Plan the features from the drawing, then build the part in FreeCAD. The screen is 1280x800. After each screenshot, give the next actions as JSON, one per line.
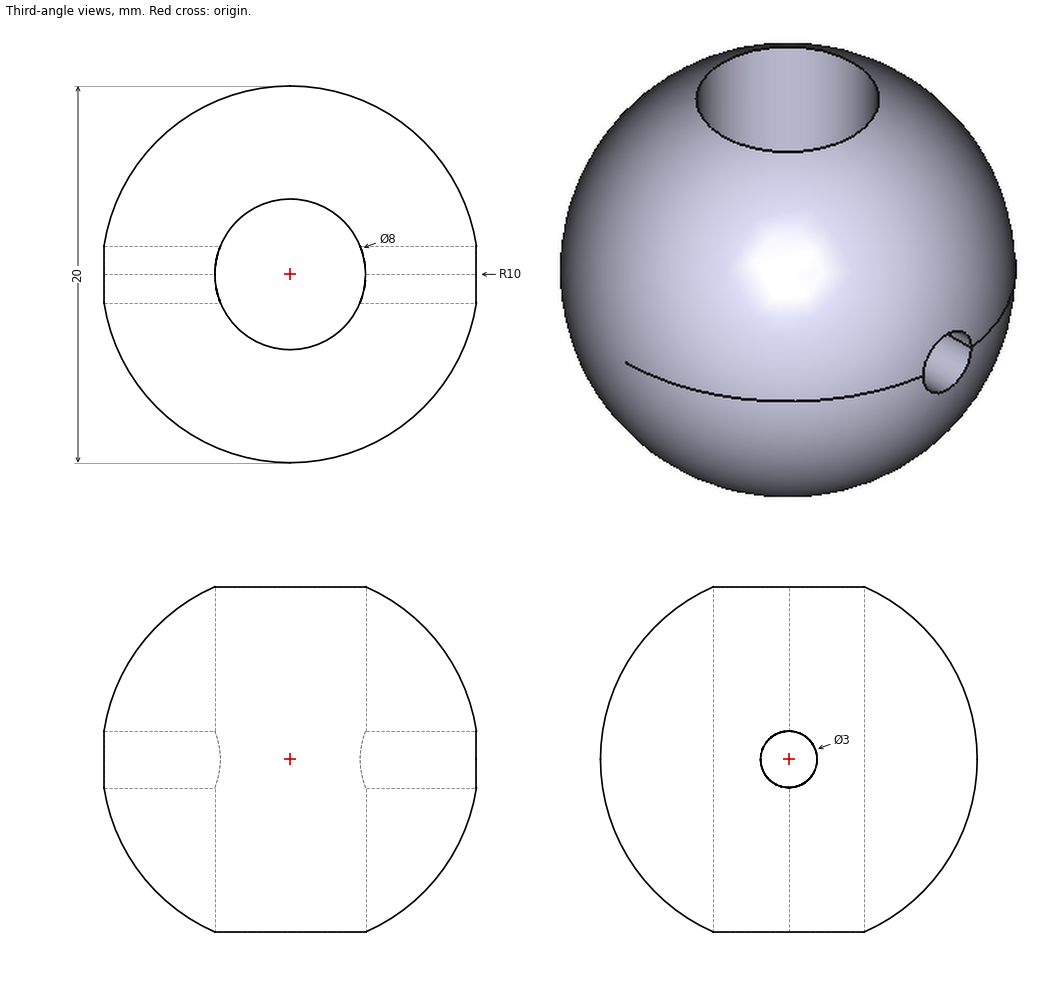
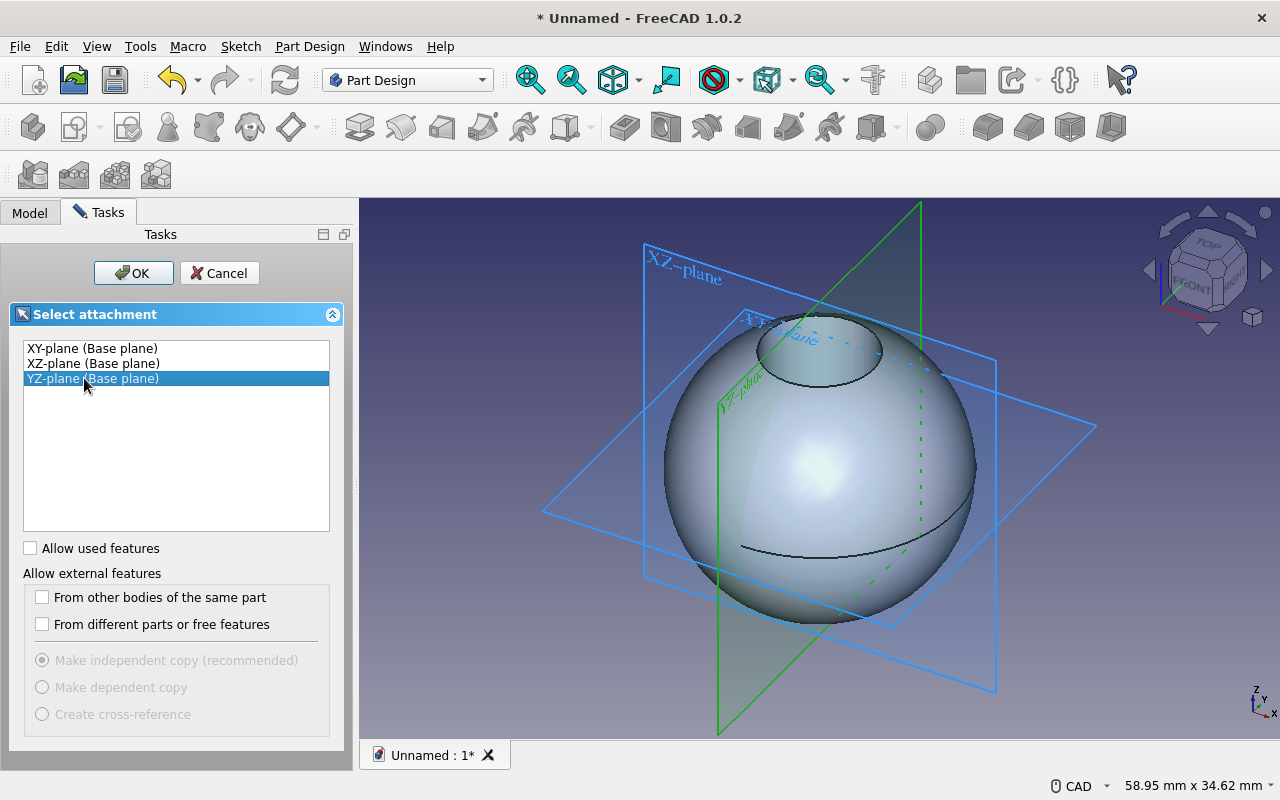
{"action": "left_click", "coordinate": [134, 273]}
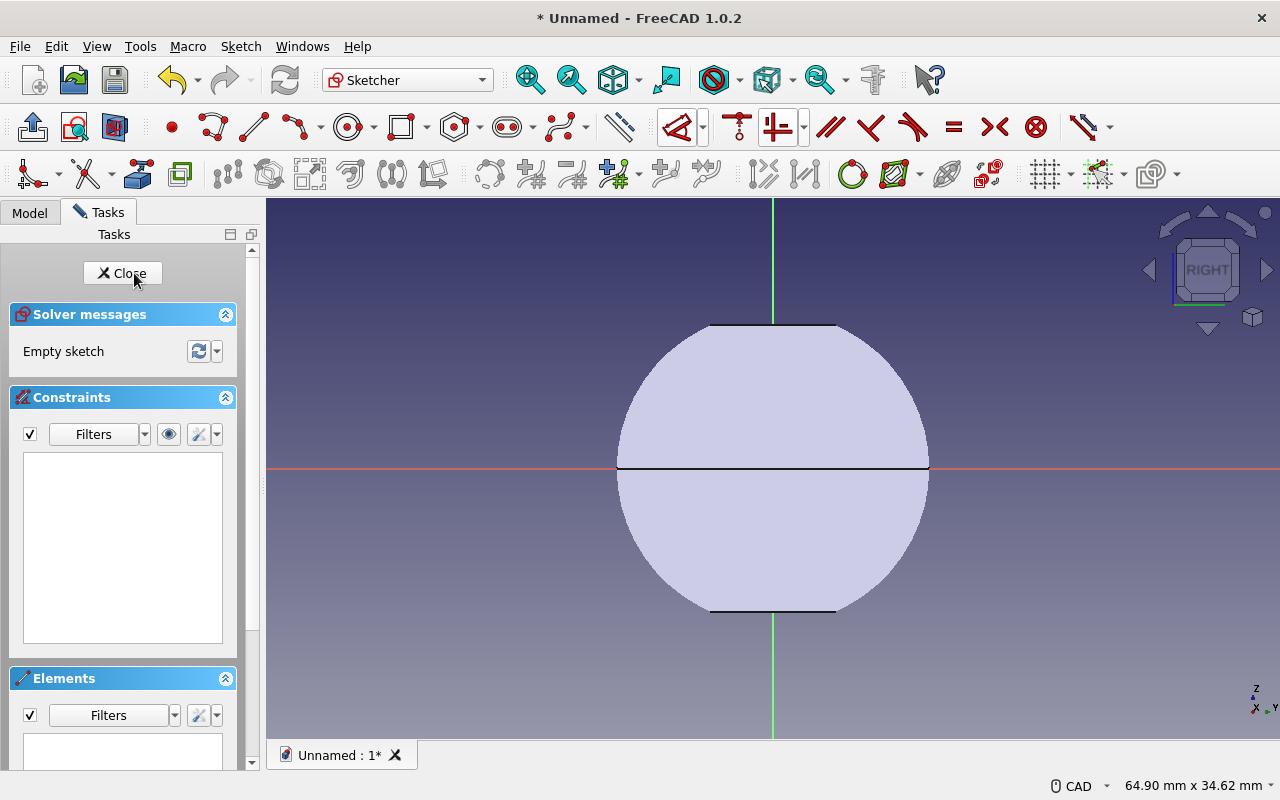
{"action": "left_click", "coordinate": [115, 128]}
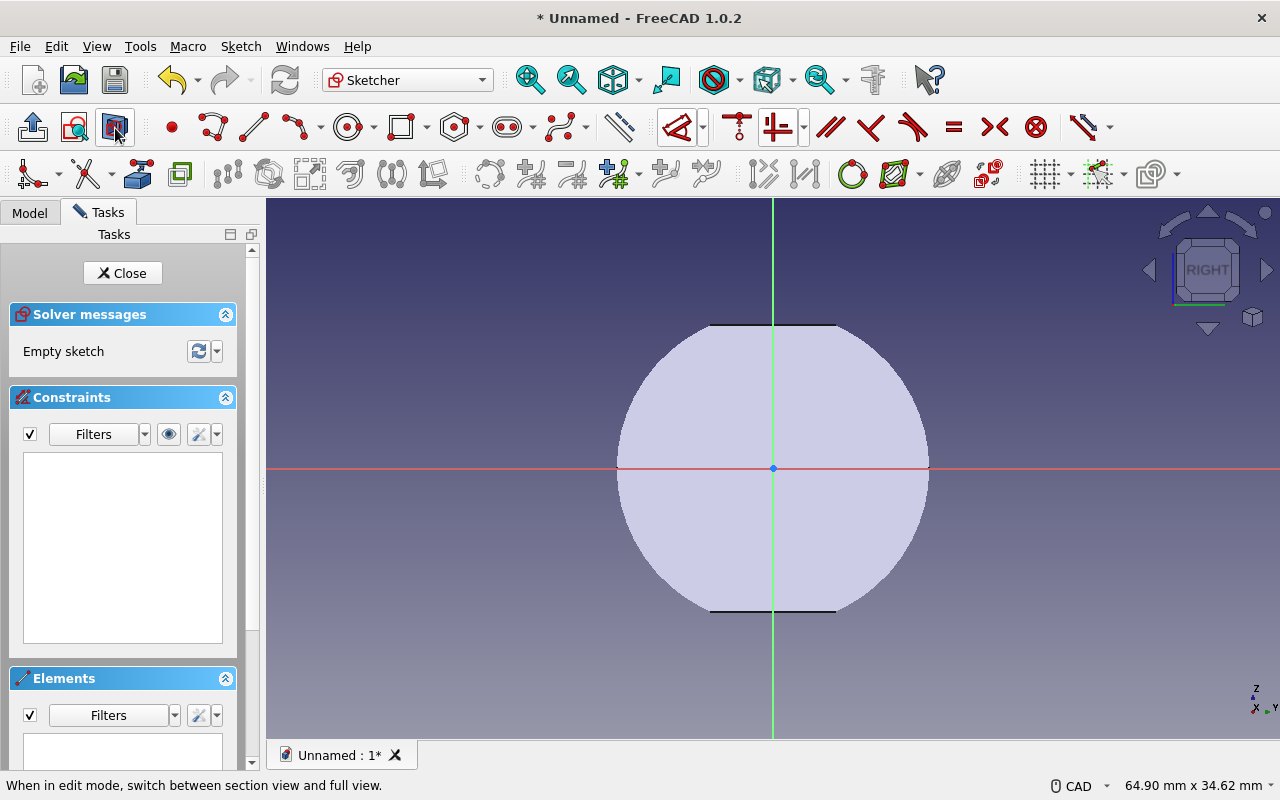
{"action": "scroll", "coordinate": [784, 468], "scroll_direction": "up", "scroll_amount": 10}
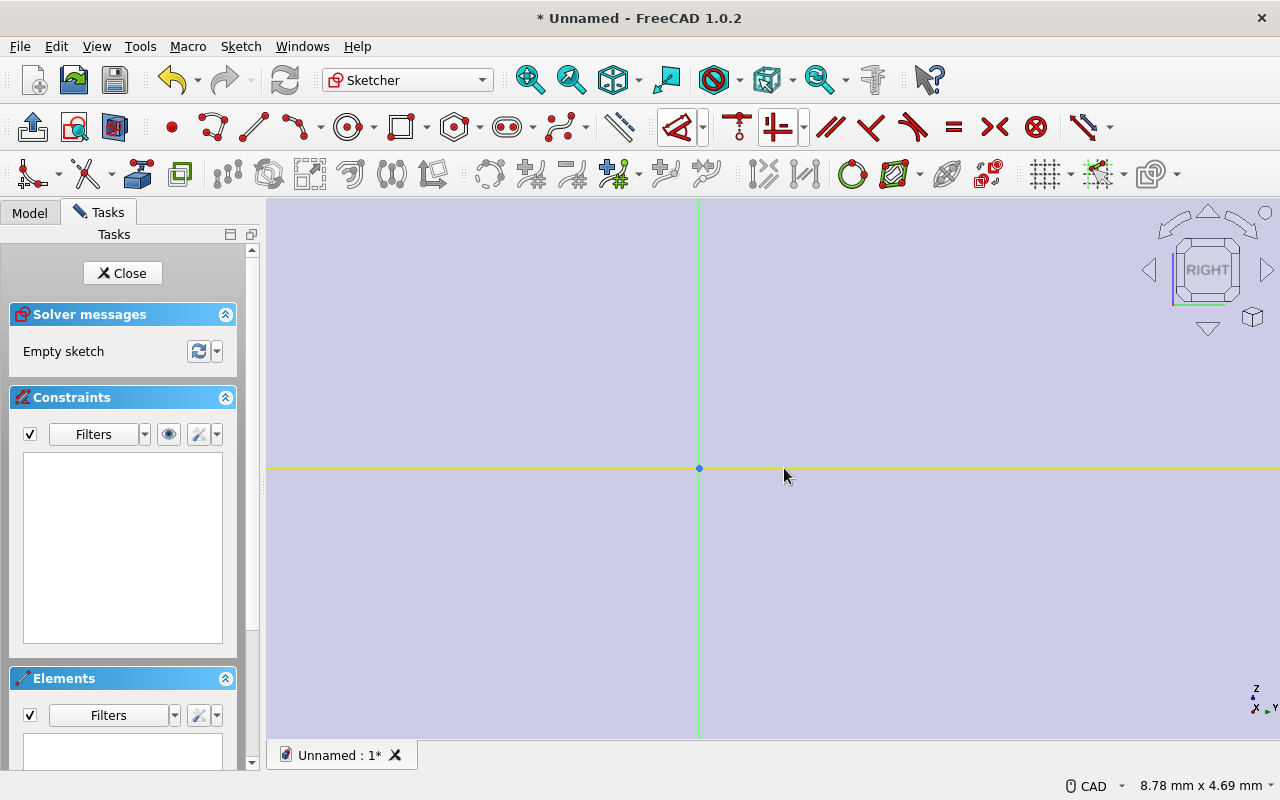
{"action": "left_click", "coordinate": [348, 128]}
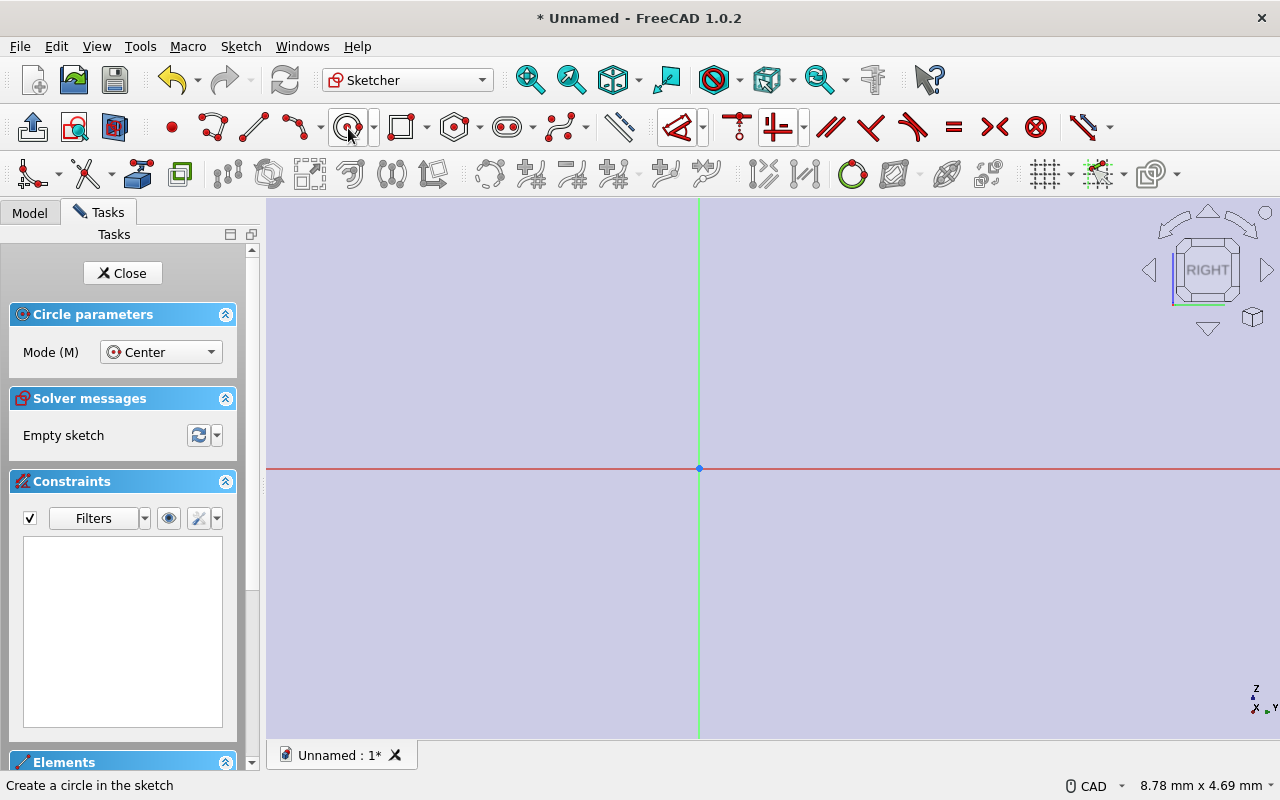
{"action": "left_click", "coordinate": [699, 468]}
{"action": "mouse_move", "coordinate": [822, 346]}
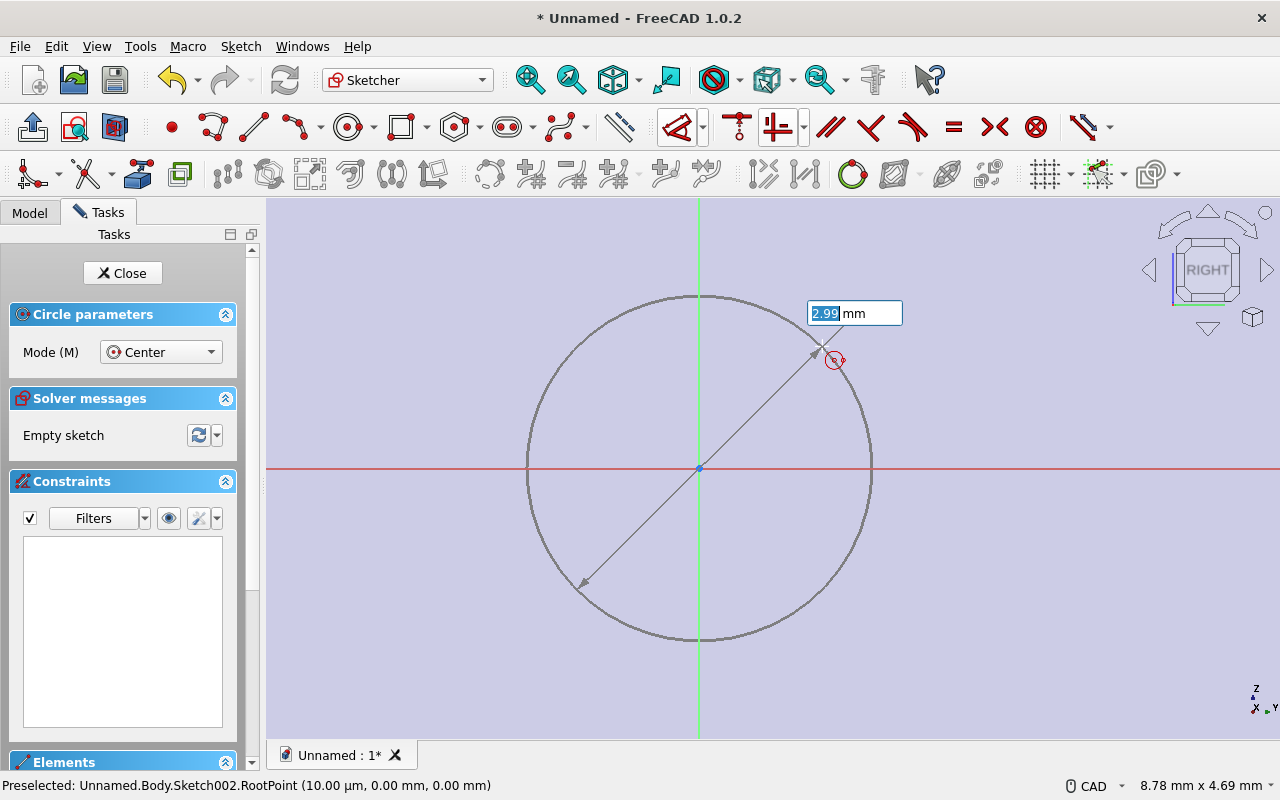
{"action": "type", "text": "3"}
{"action": "key", "text": "Return"}
{"action": "key", "text": "Escape"}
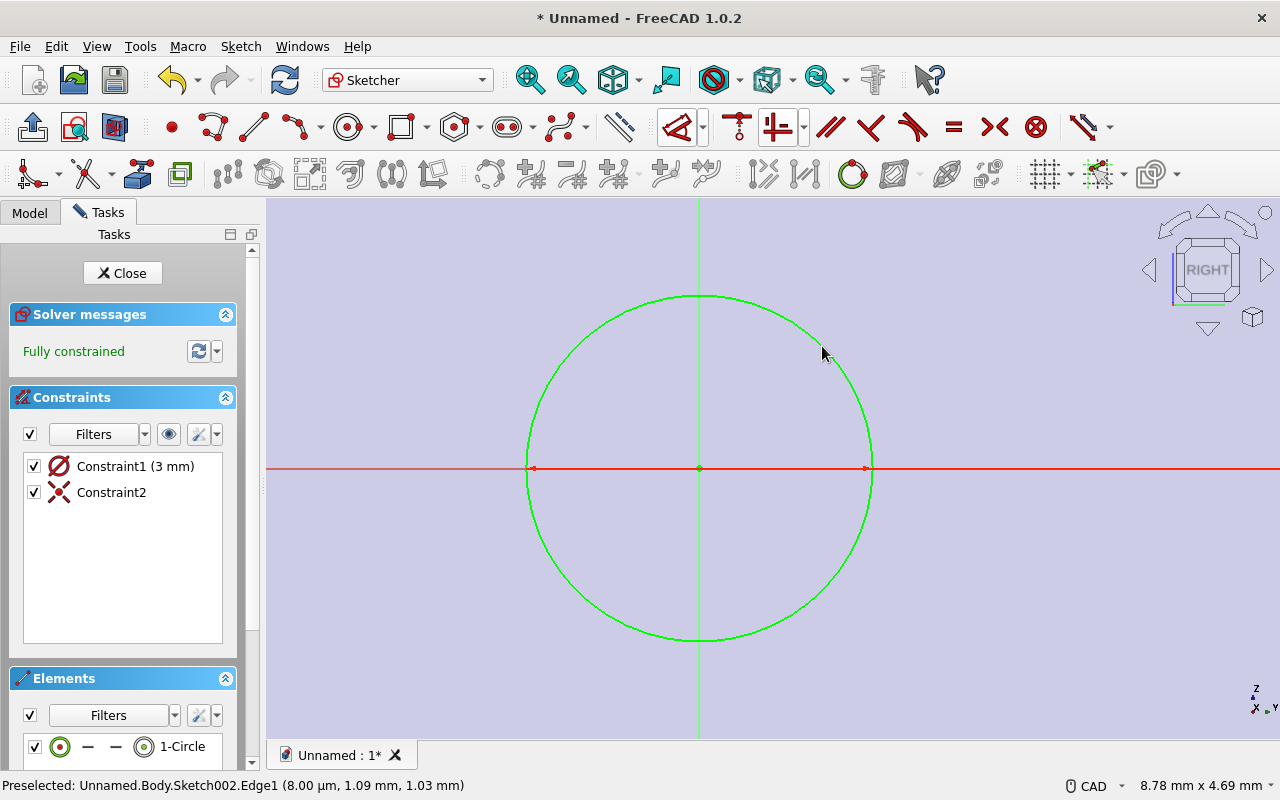
{"action": "left_click", "coordinate": [123, 273]}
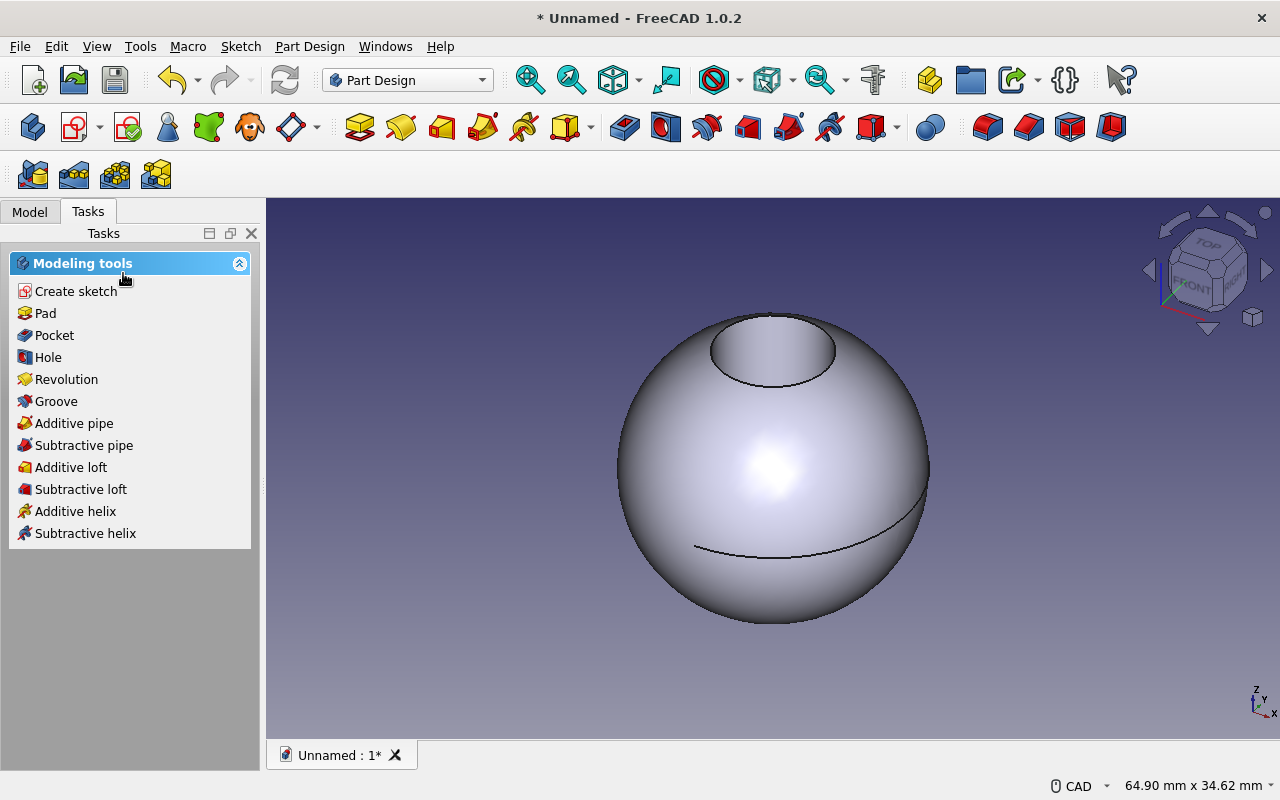
{"action": "left_click", "coordinate": [625, 128]}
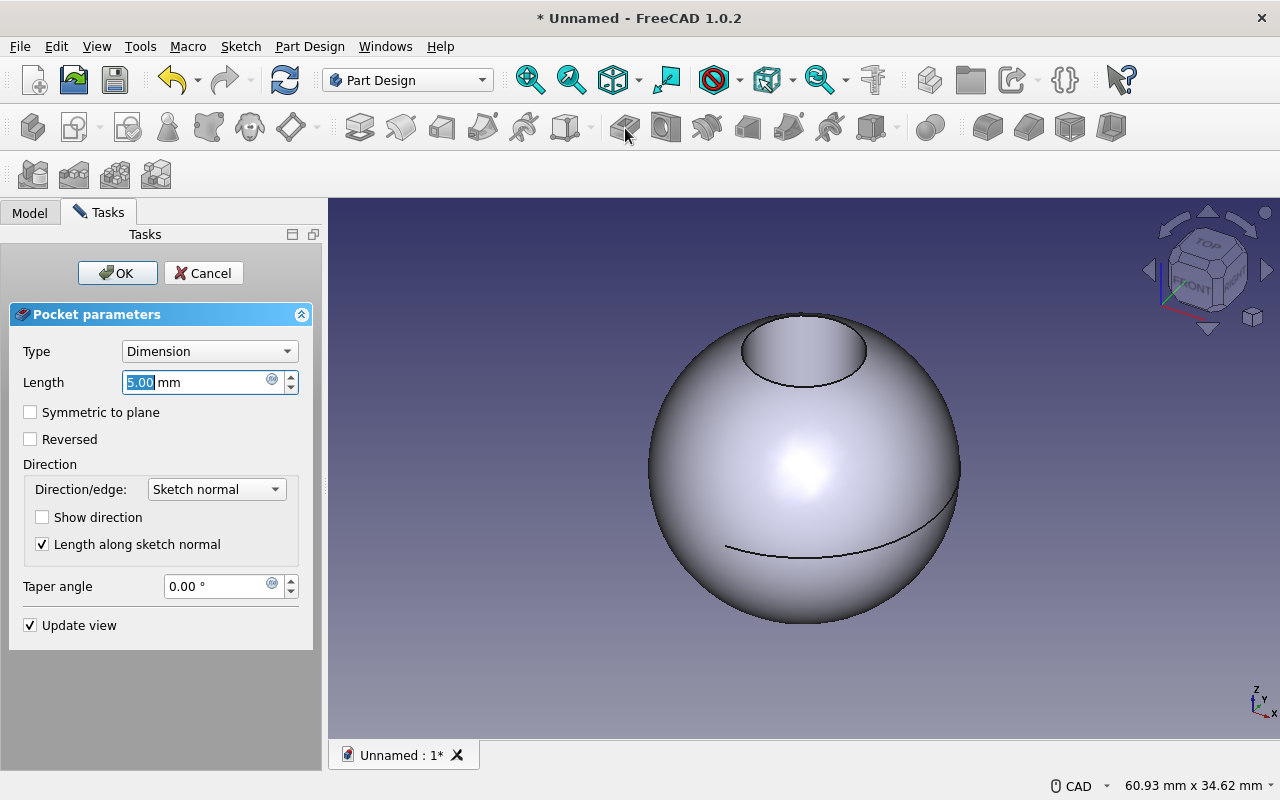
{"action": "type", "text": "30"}
{"action": "key", "text": "Tab"}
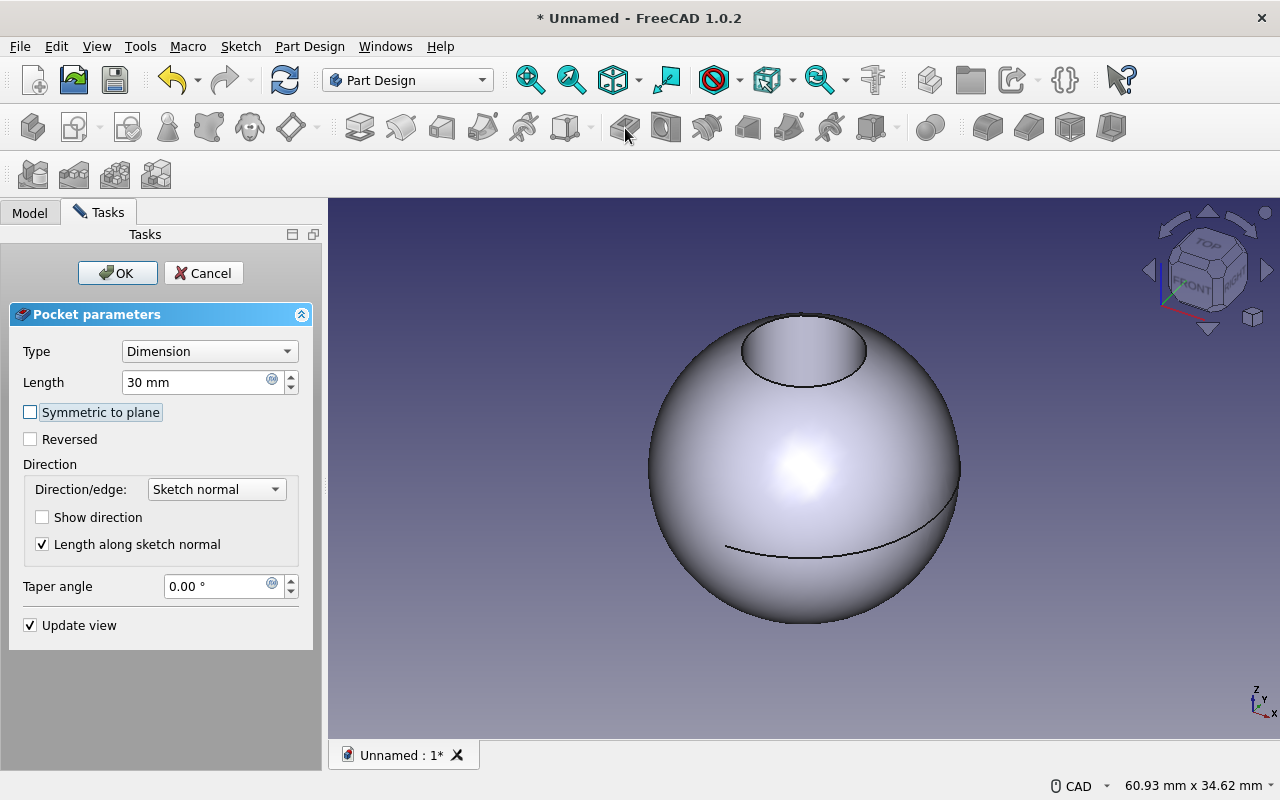
{"action": "left_click", "coordinate": [31, 412]}